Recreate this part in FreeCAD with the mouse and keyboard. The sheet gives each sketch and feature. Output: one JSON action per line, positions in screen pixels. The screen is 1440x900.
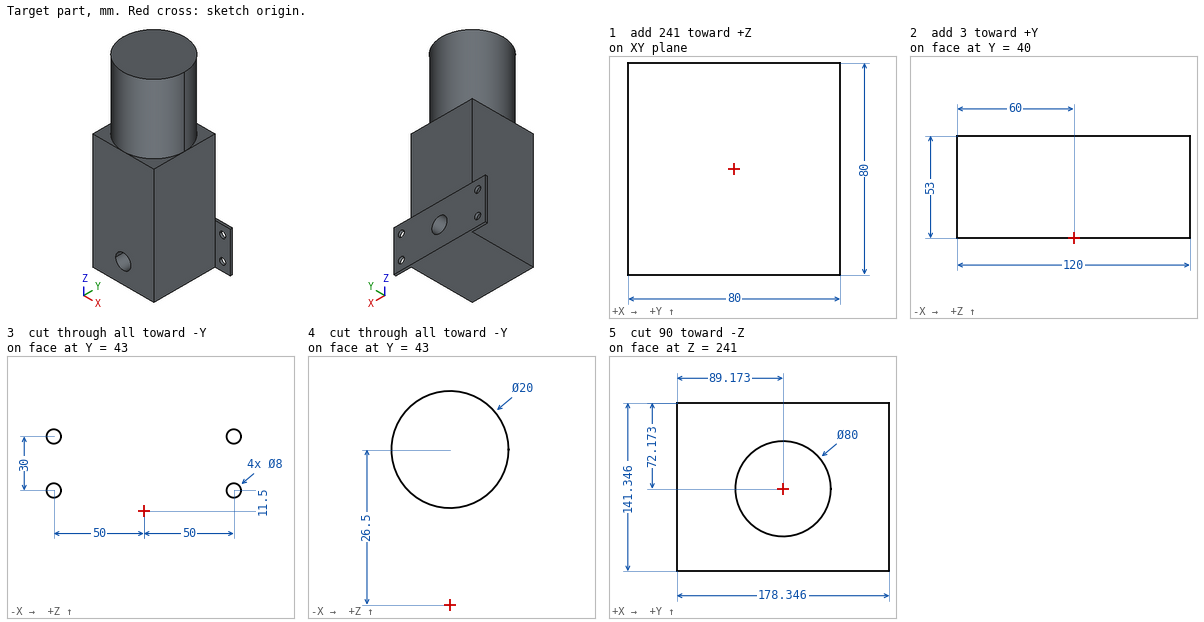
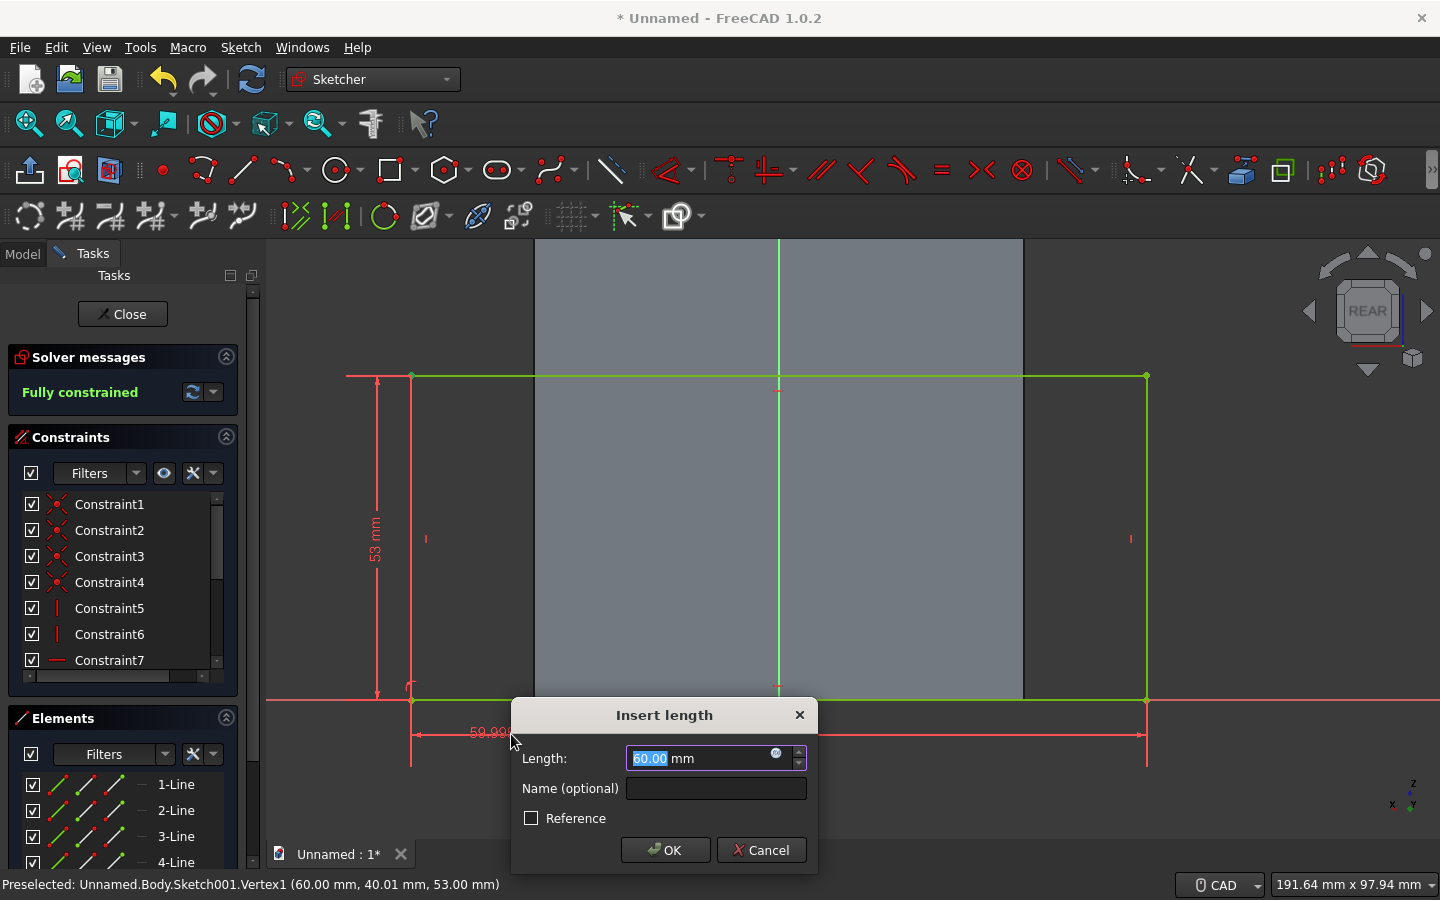
{"action": "type", "text": "60"}
{"action": "key", "text": "Return"}
{"action": "key", "text": "Escape"}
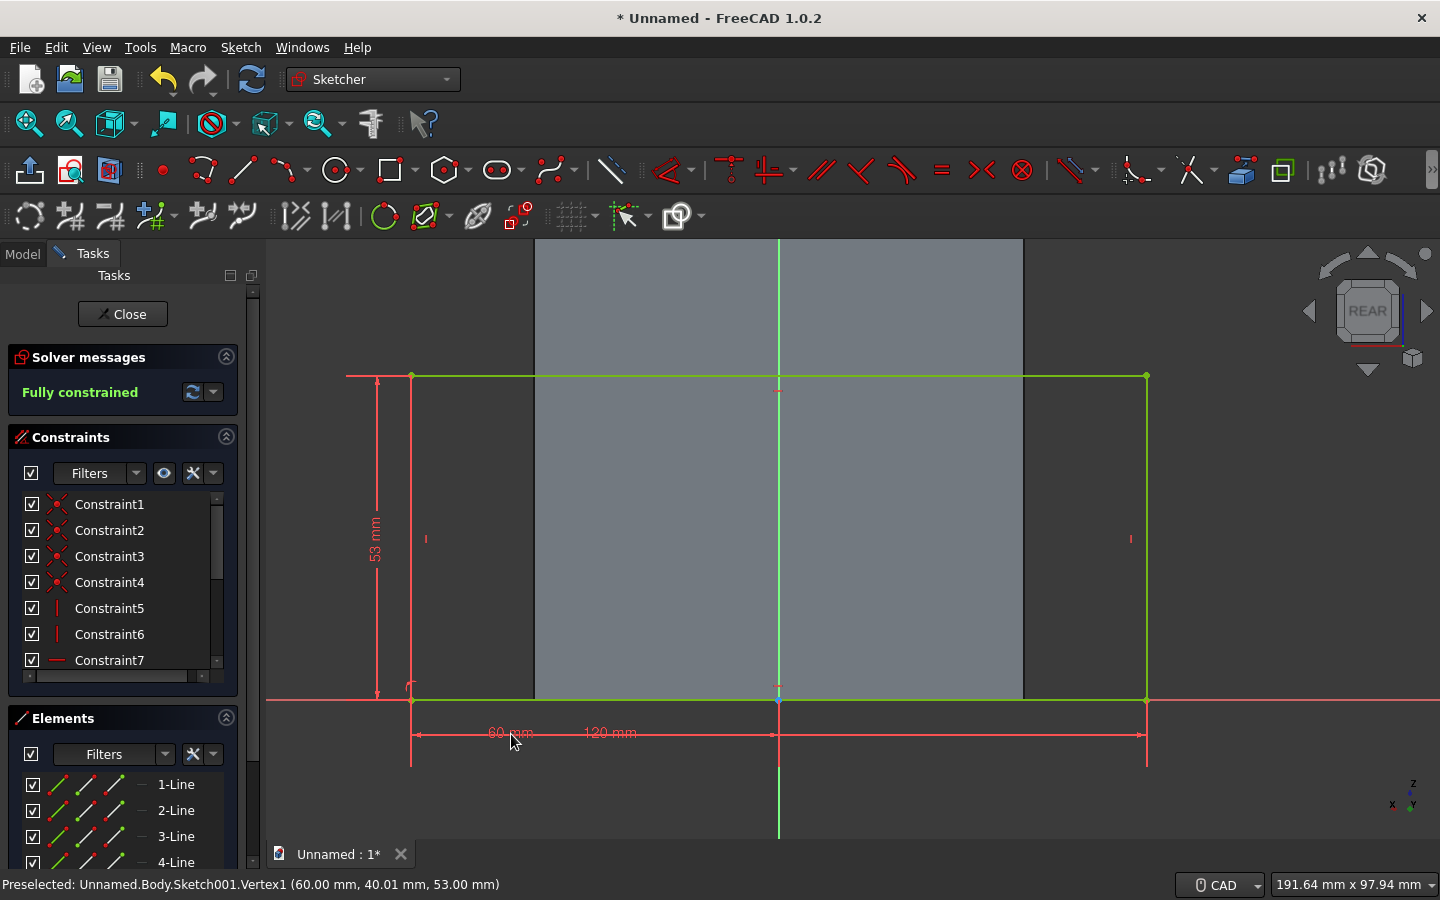
{"action": "left_click", "coordinate": [123, 314]}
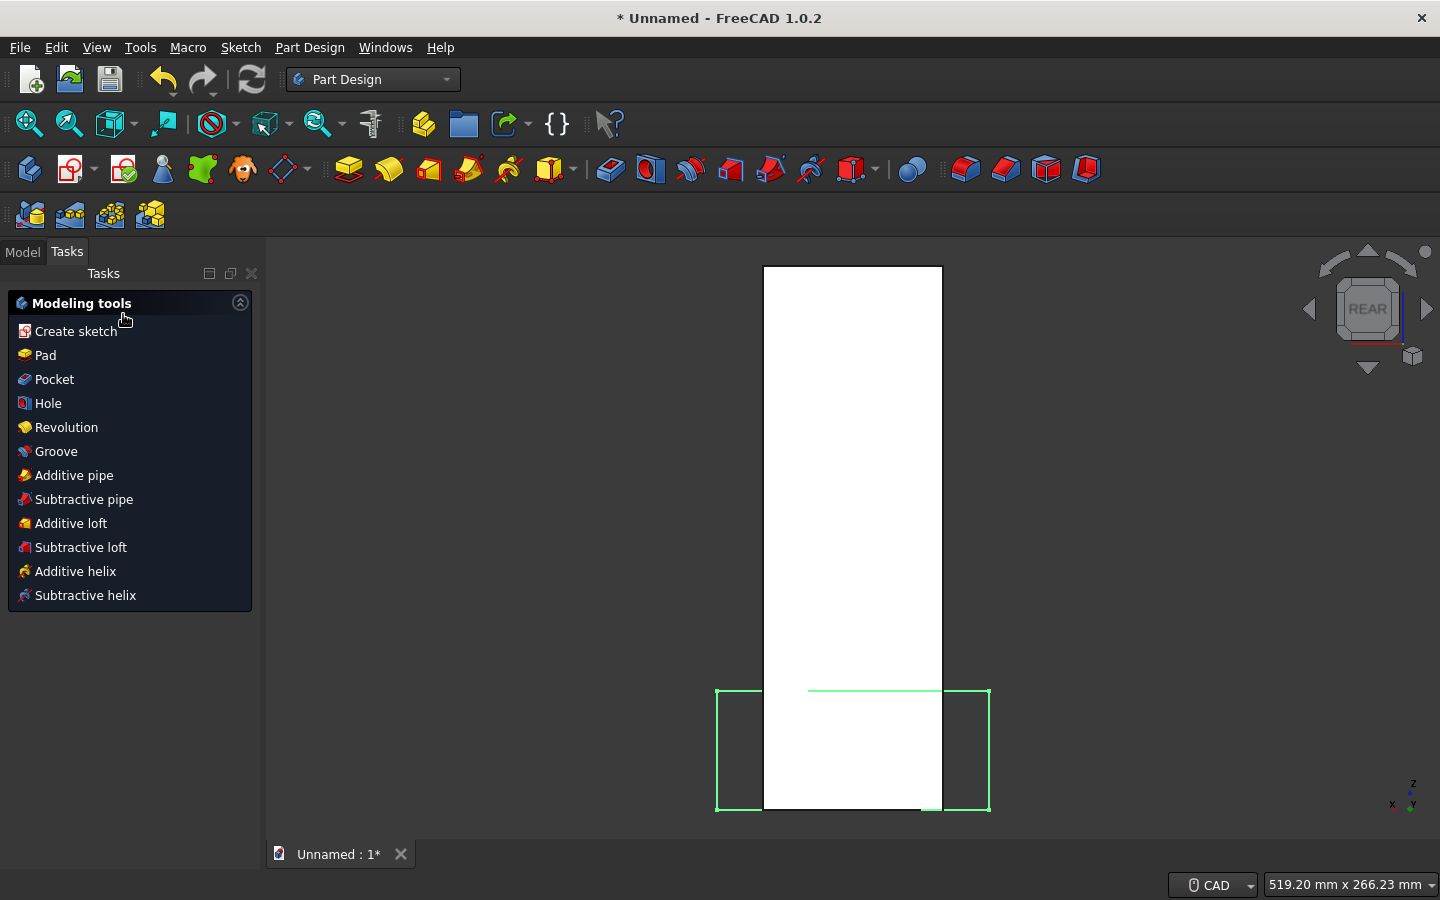
{"action": "left_click", "coordinate": [350, 170]}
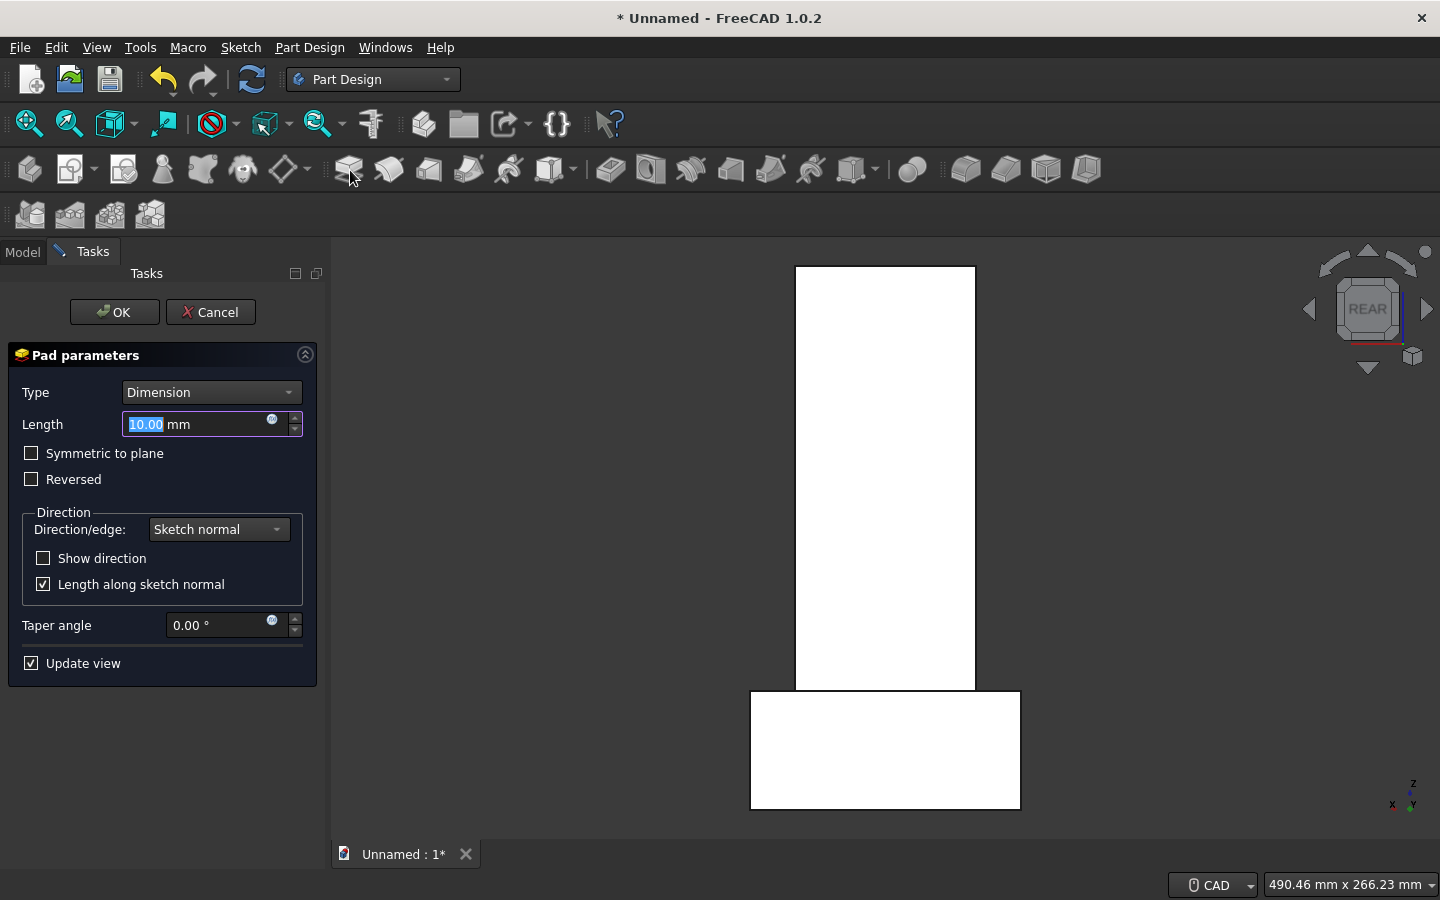
{"action": "type", "text": "3"}
{"action": "key", "text": "Tab"}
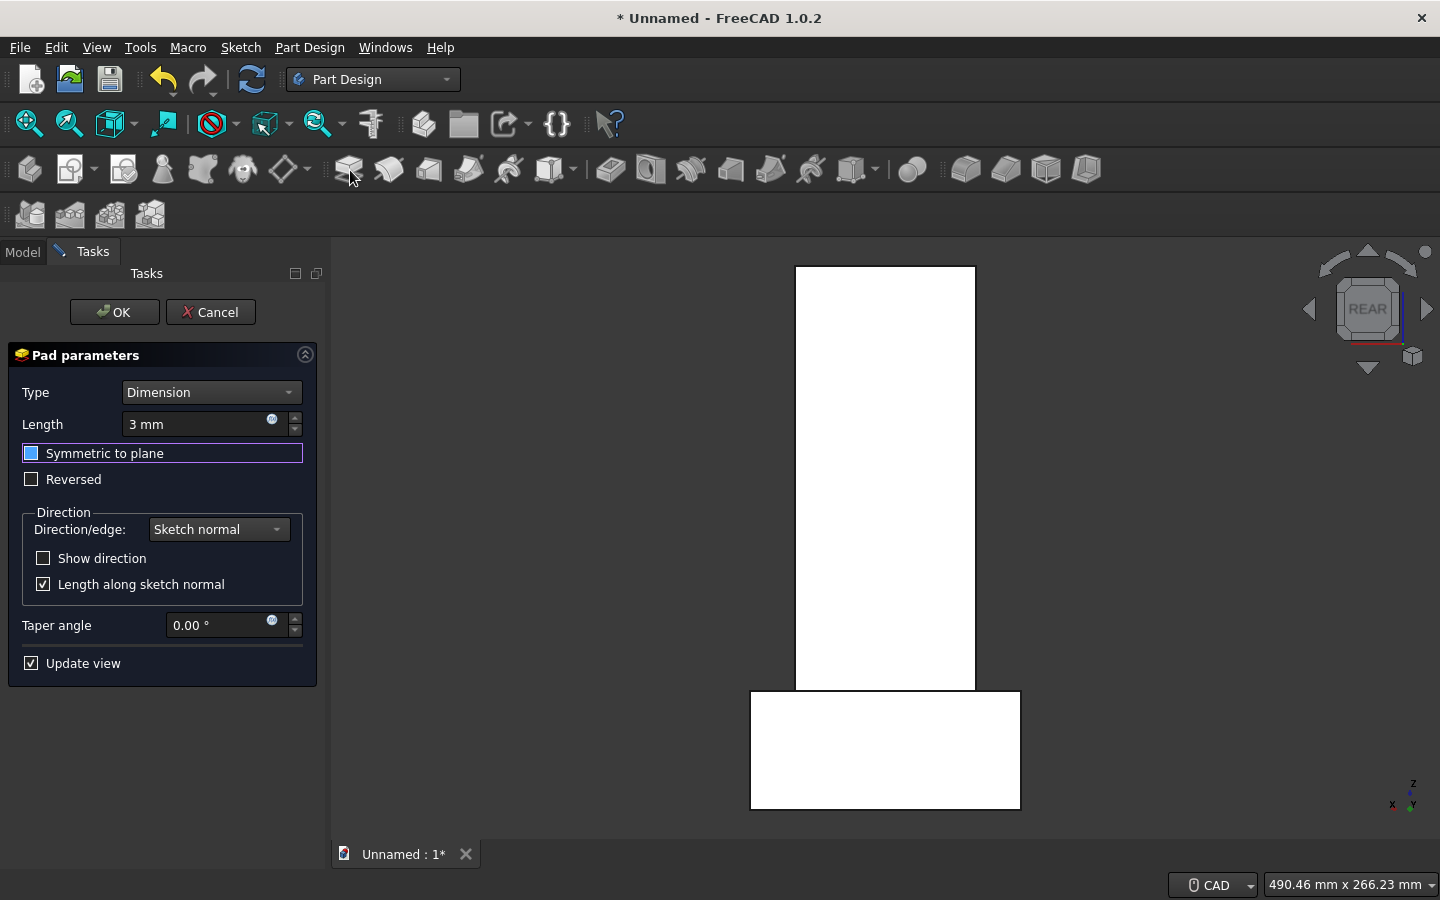
{"action": "left_click", "coordinate": [115, 312]}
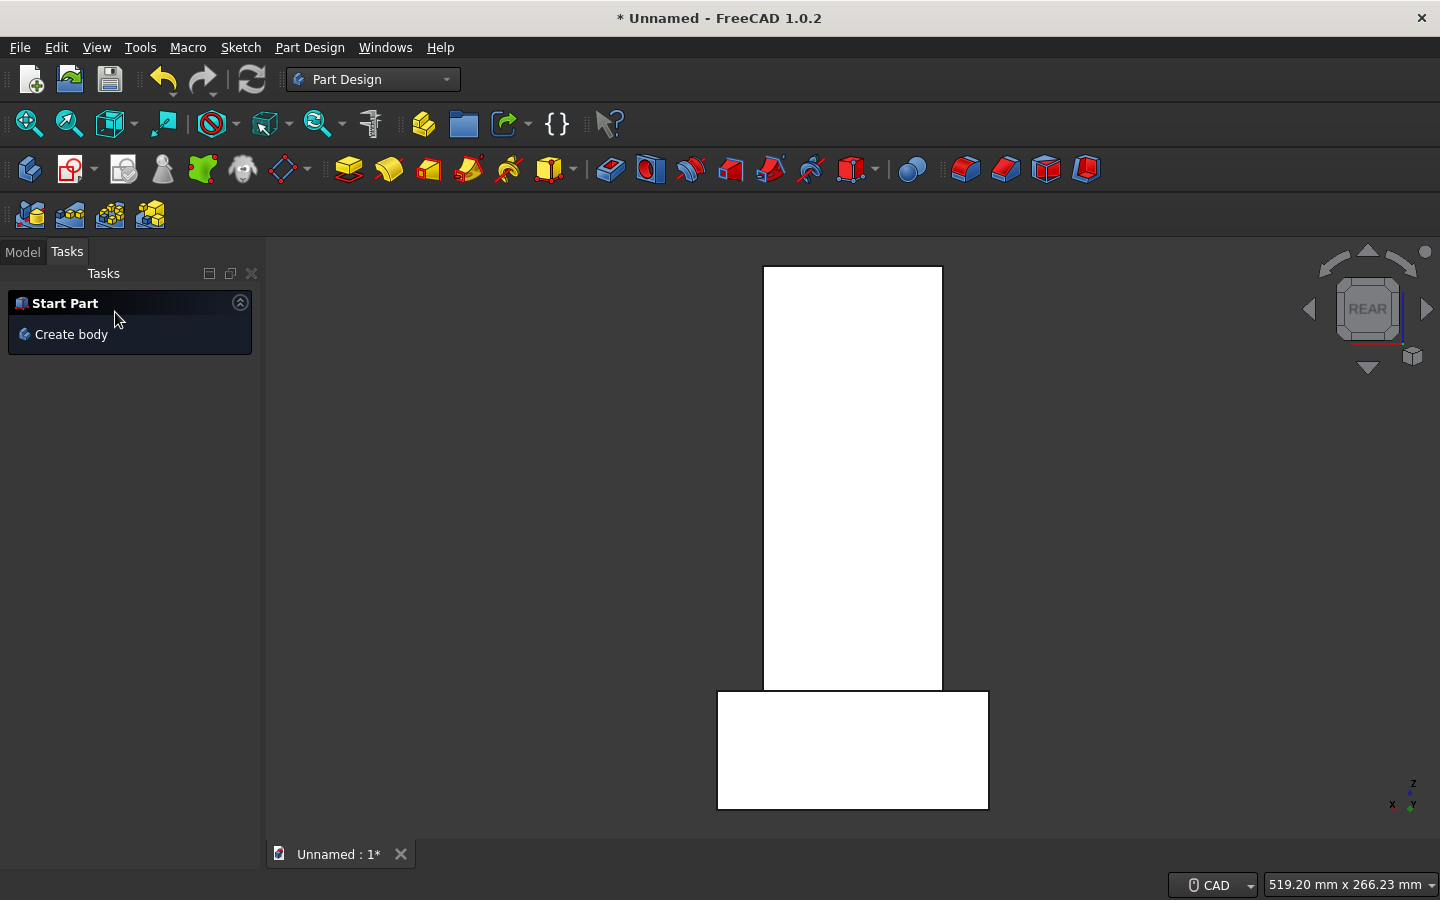
{"action": "left_click", "coordinate": [814, 750]}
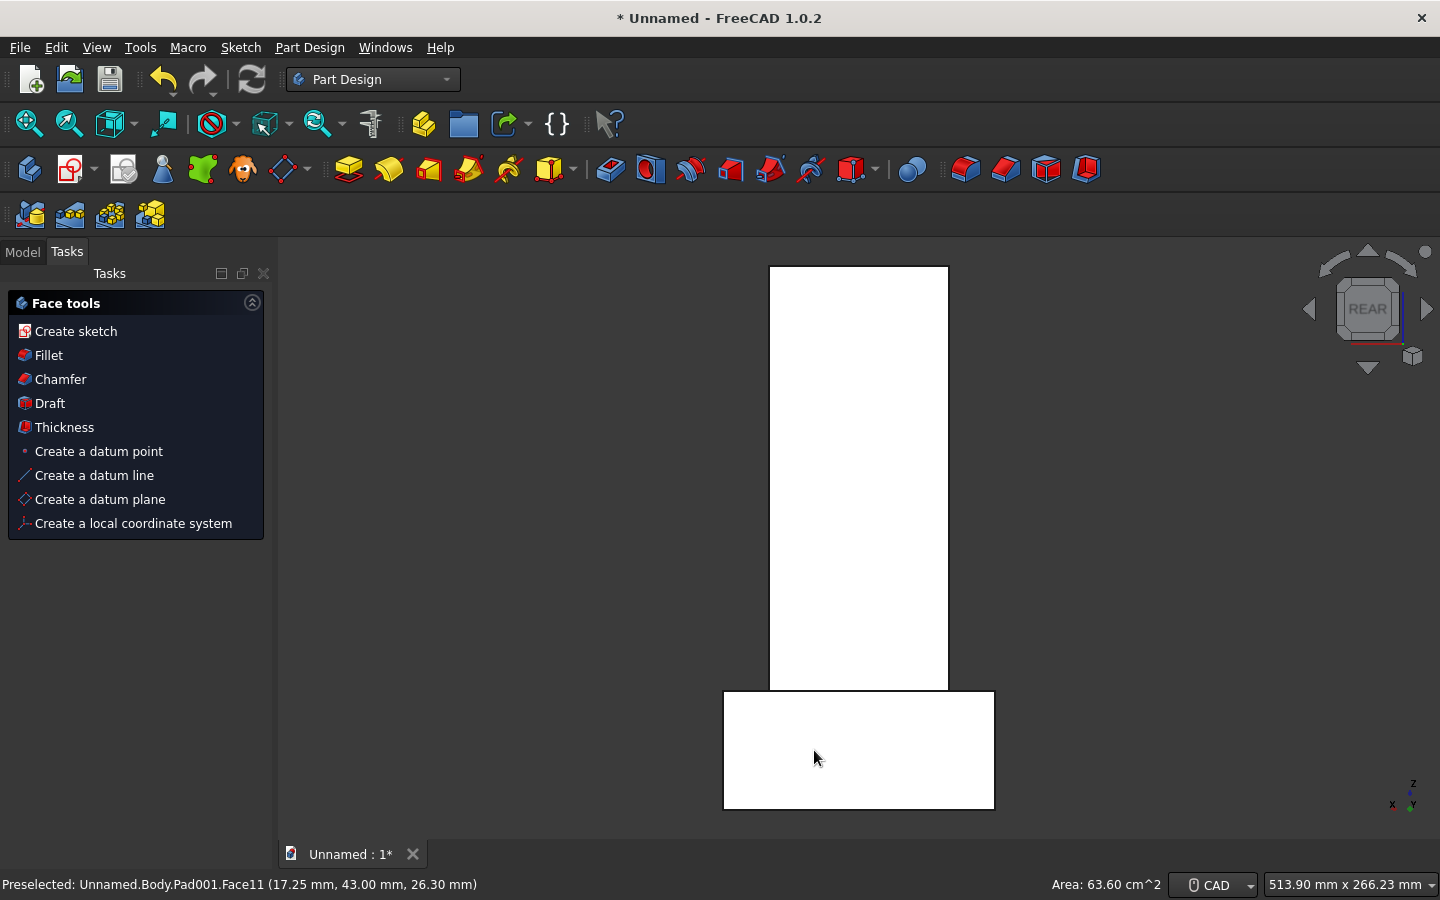
{"action": "left_click", "coordinate": [70, 170]}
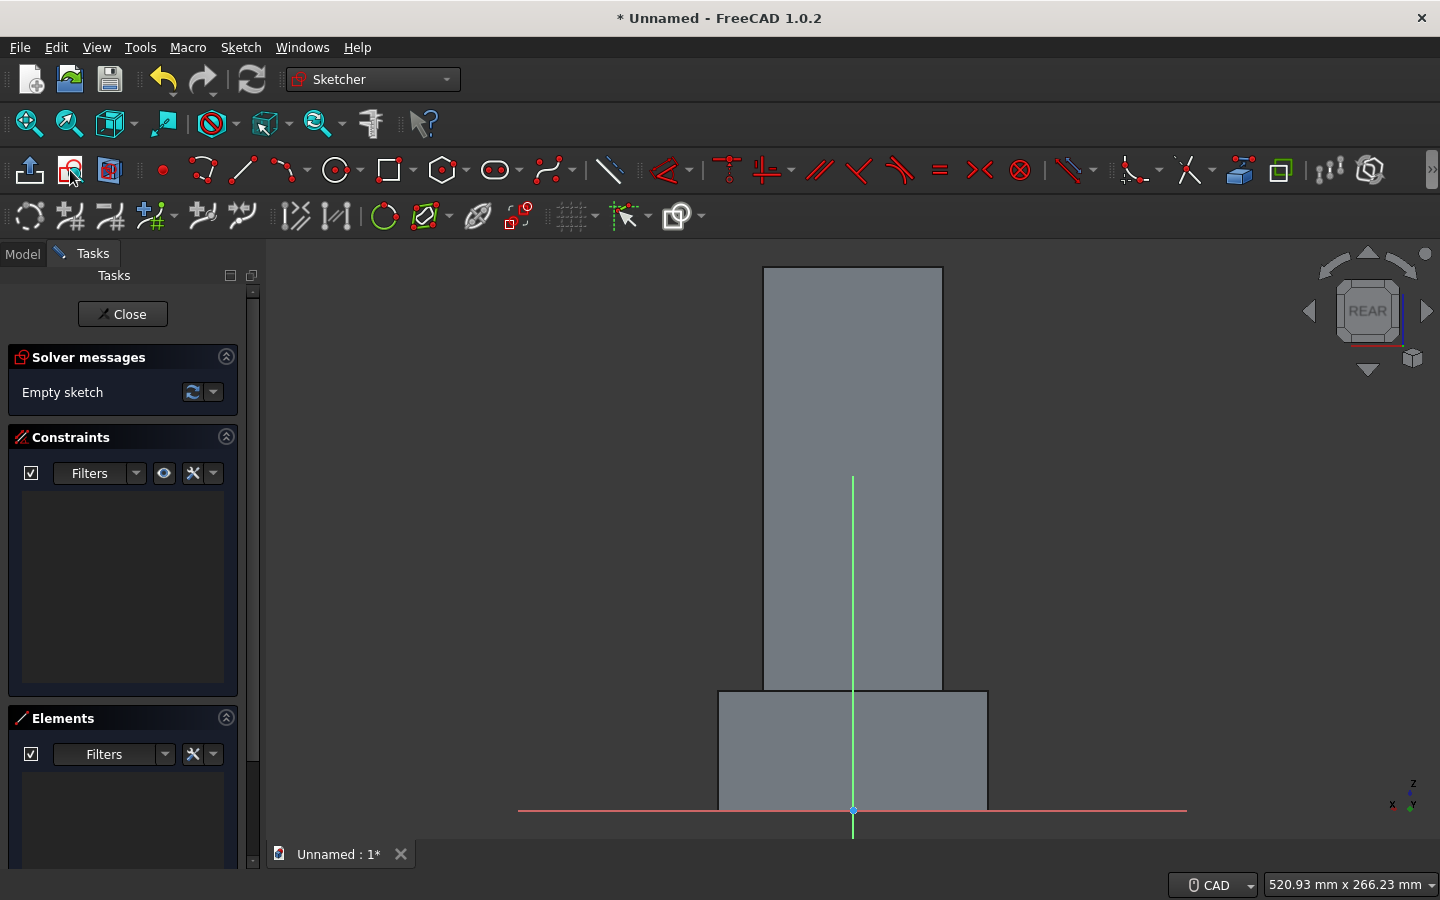
{"action": "scroll", "coordinate": [784, 539], "scroll_direction": "down", "scroll_amount": 5}